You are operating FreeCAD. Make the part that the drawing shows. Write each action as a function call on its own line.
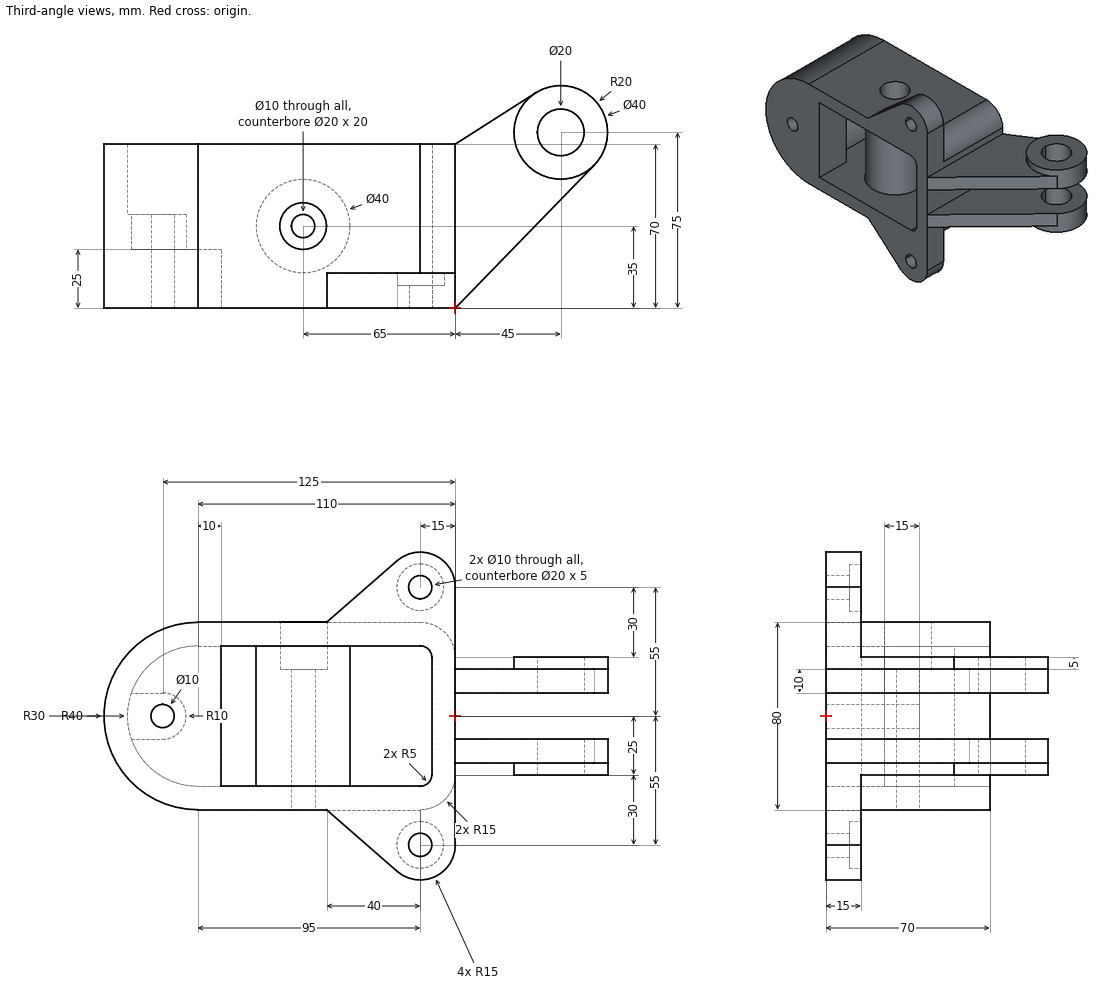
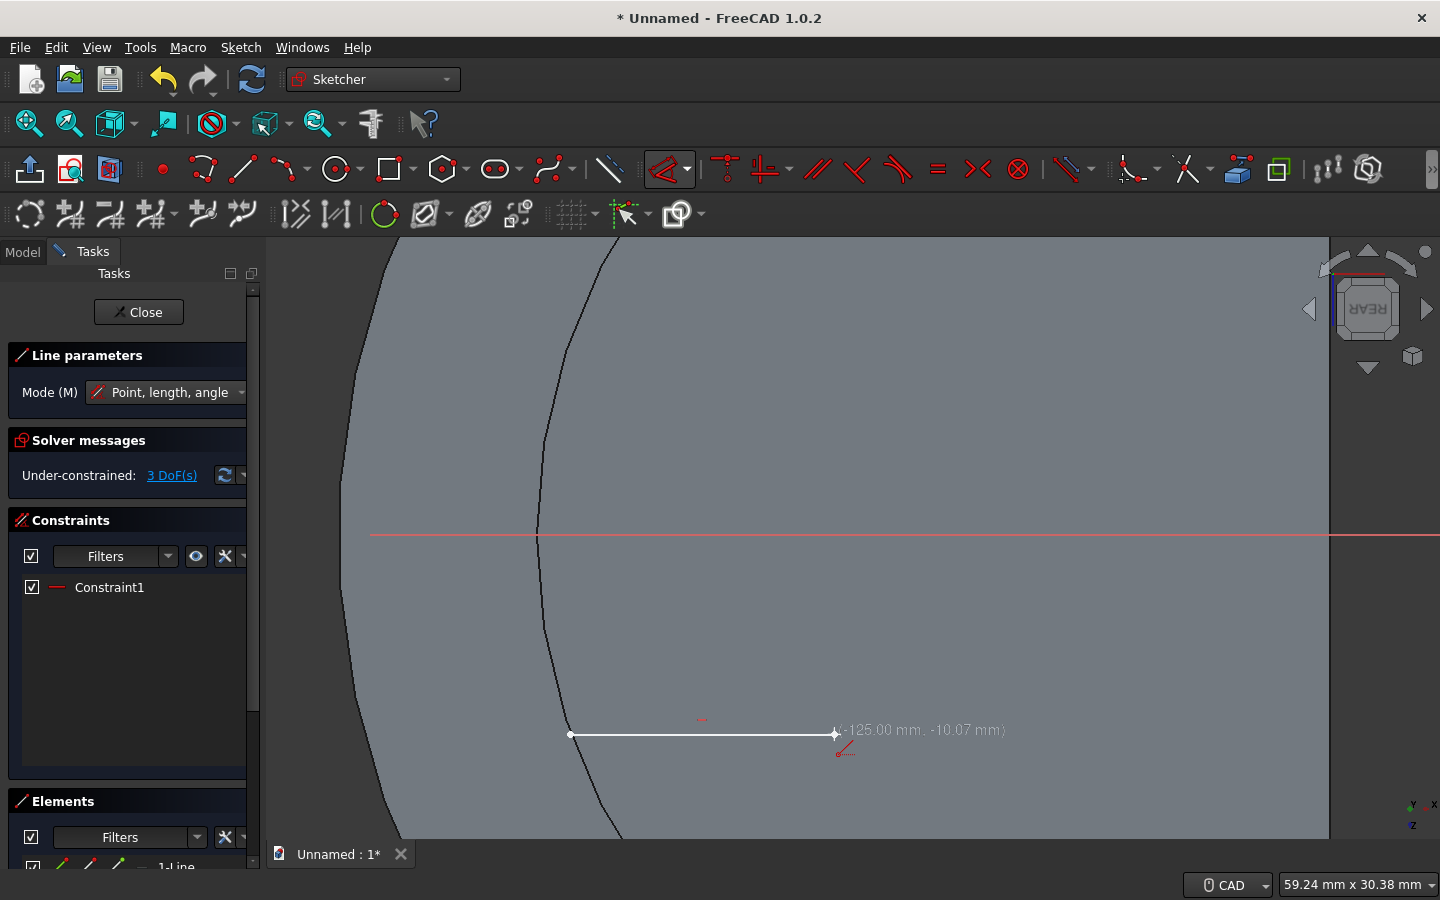
click(834, 337)
click(571, 337)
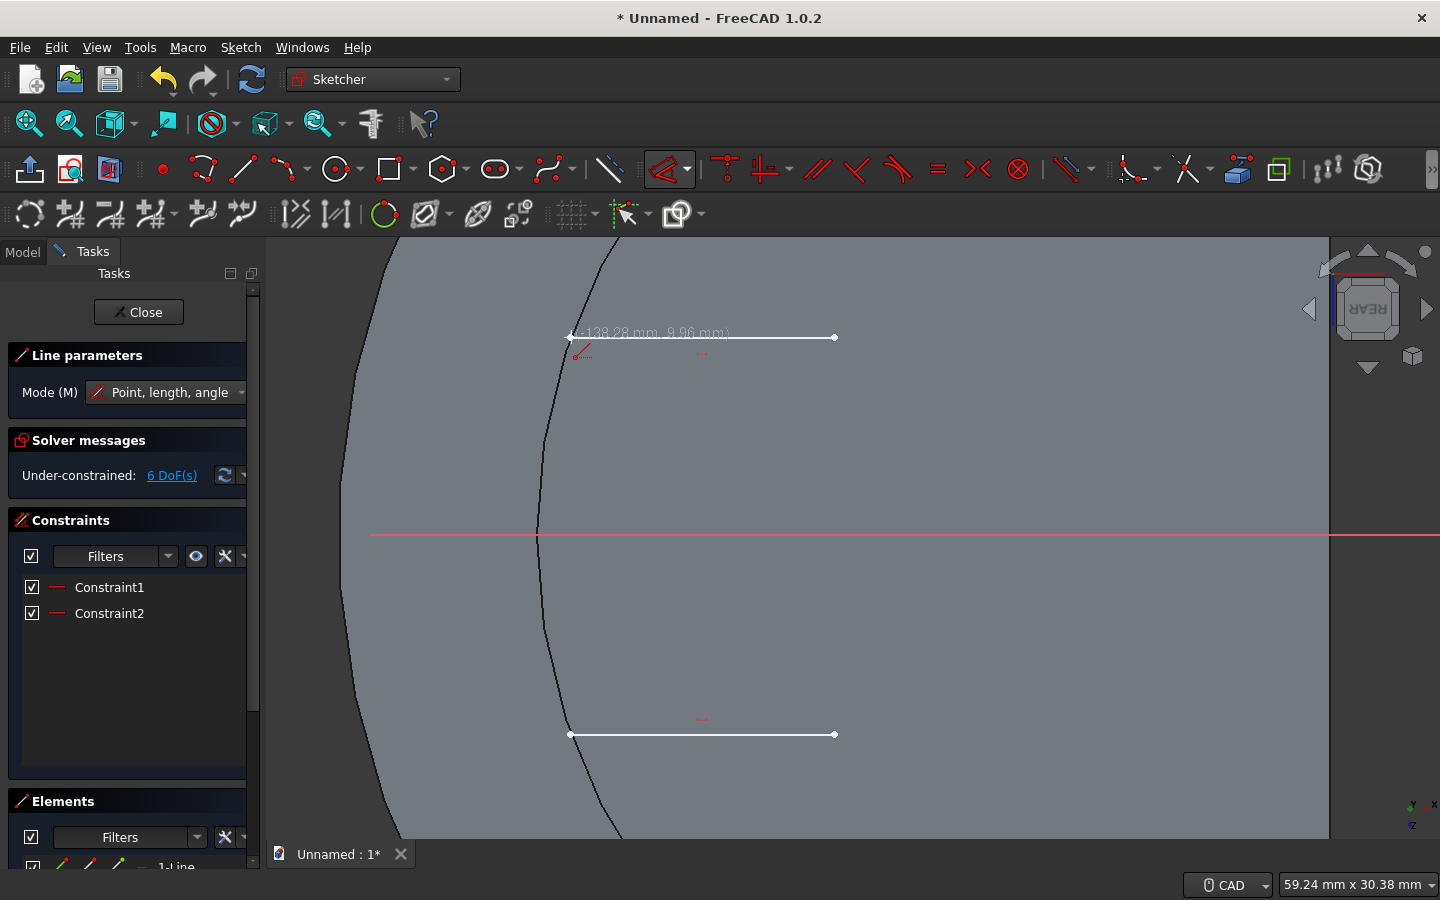
key(g)
key(3)
key(a)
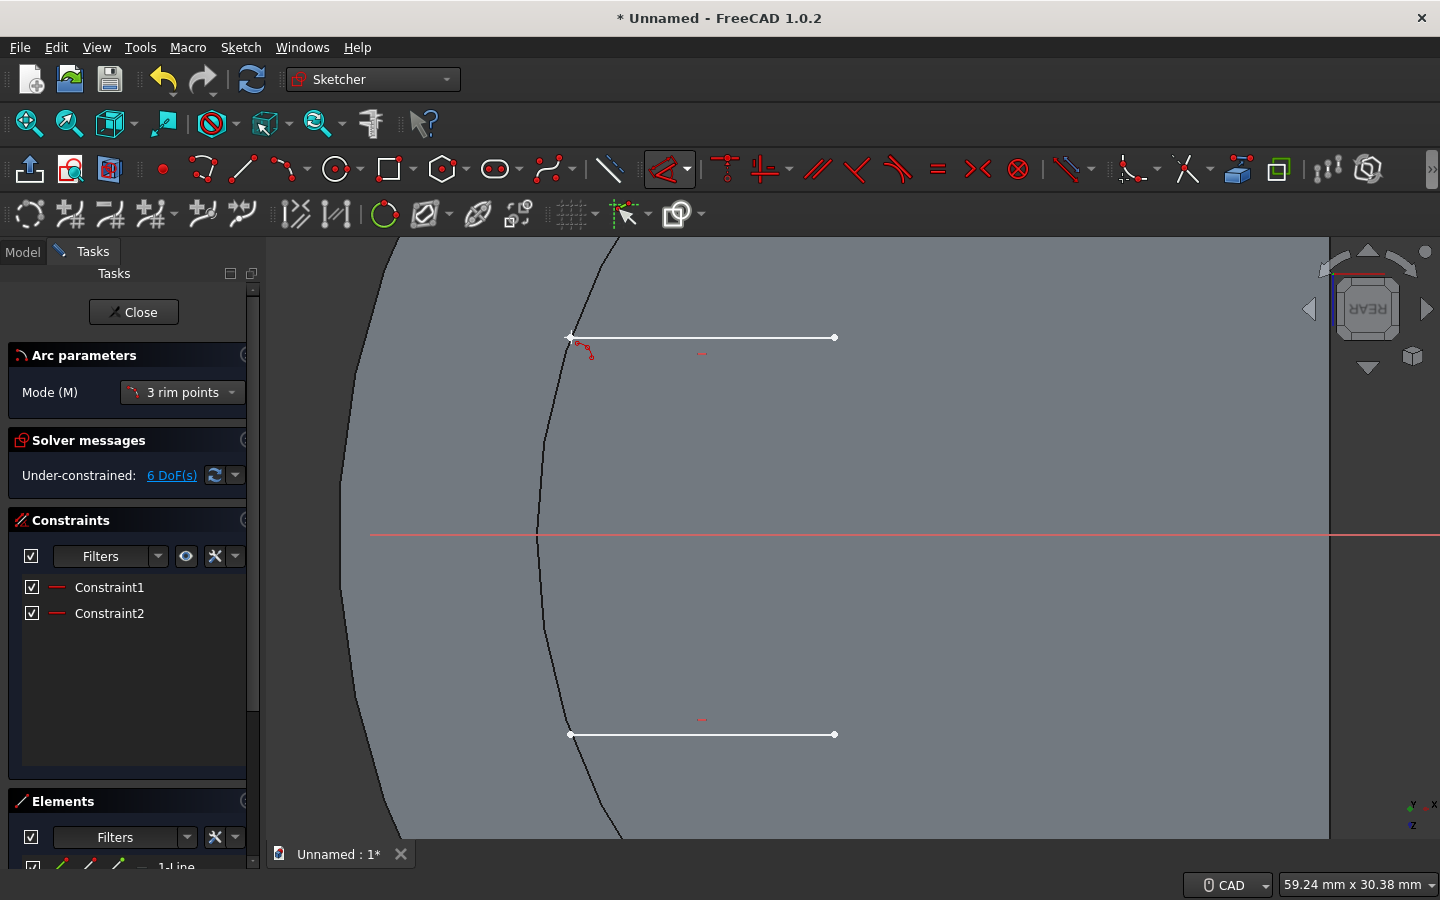
click(834, 735)
click(834, 338)
click(1023, 597)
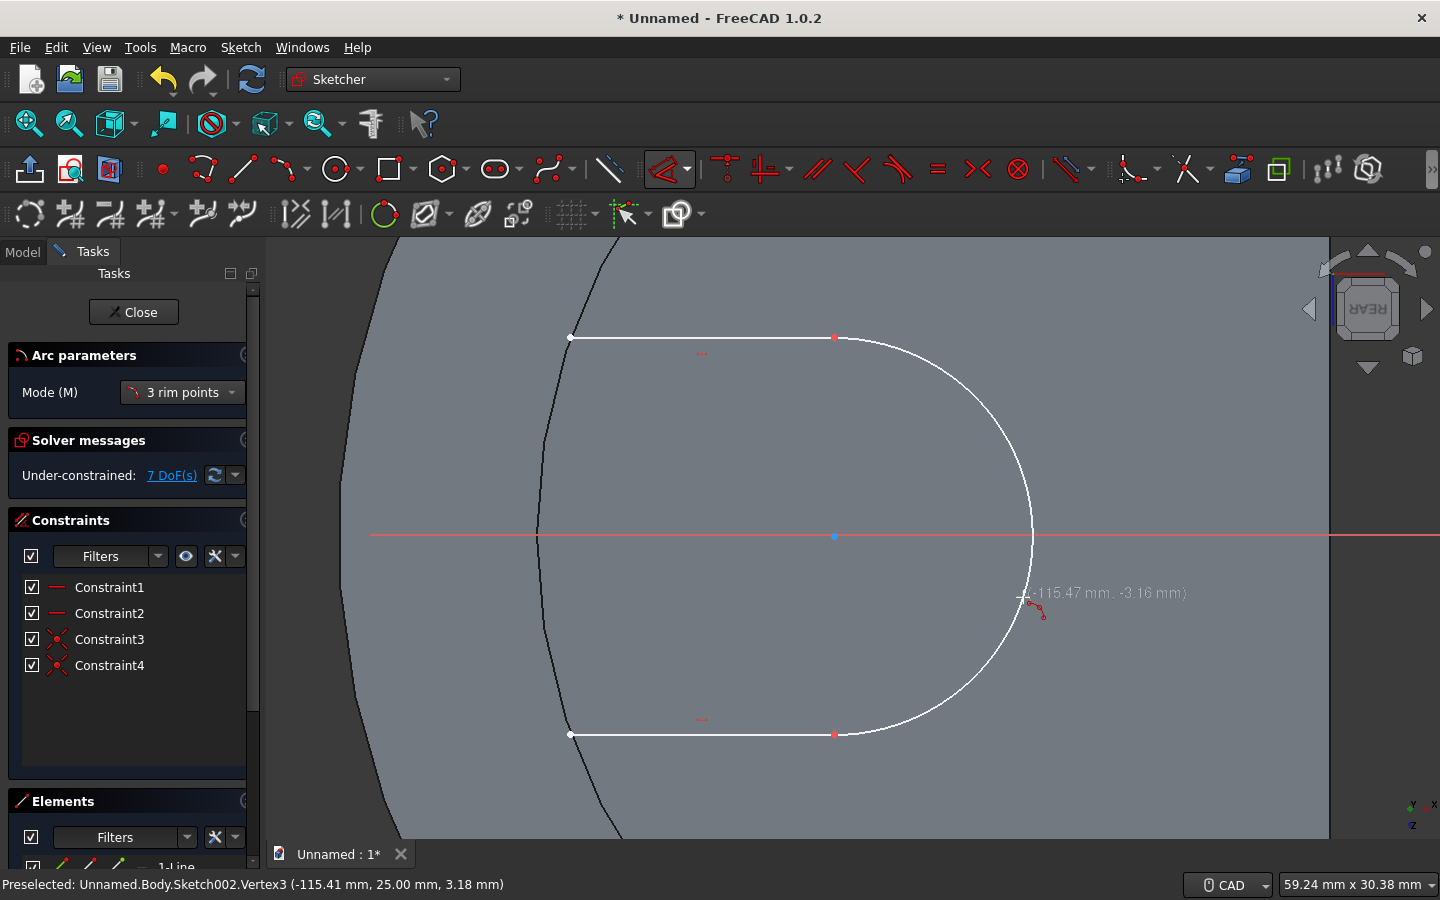
click(571, 338)
click(571, 735)
click(538, 495)
key(Escape)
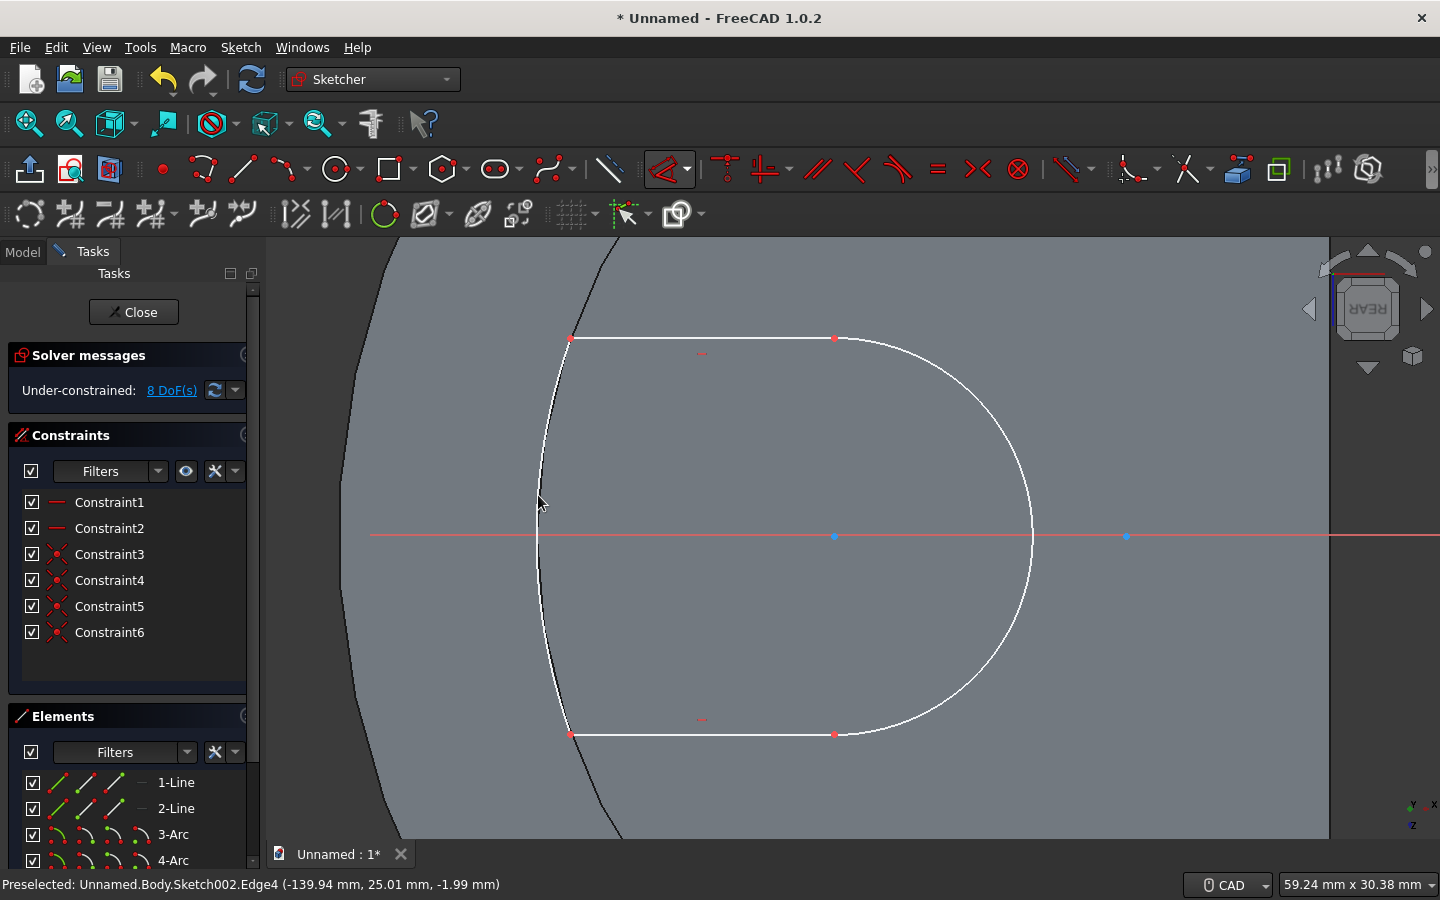
click(650, 735)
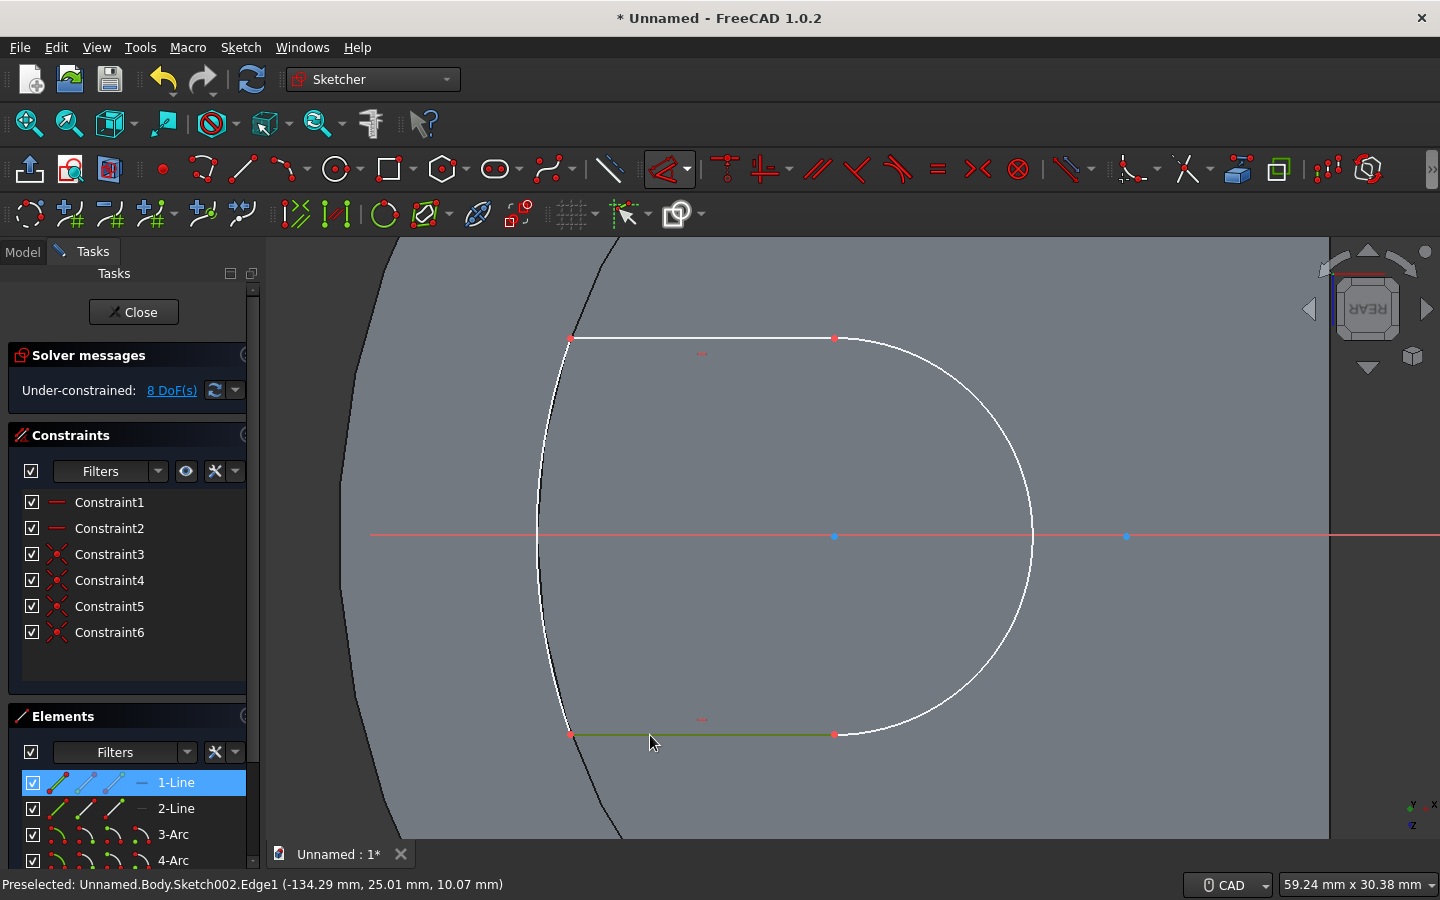
click(995, 653)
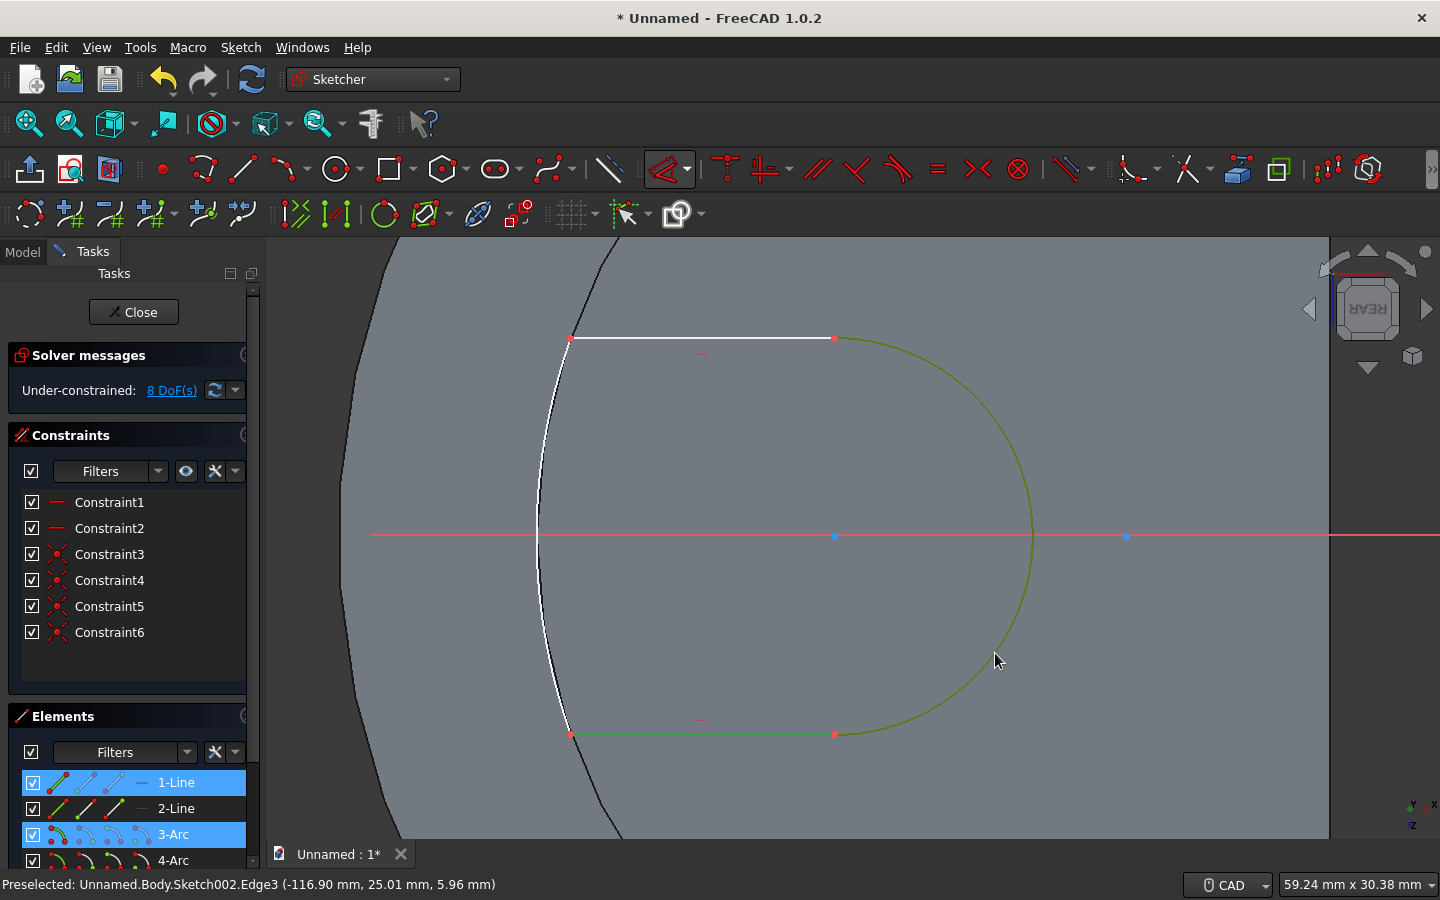
key(t)